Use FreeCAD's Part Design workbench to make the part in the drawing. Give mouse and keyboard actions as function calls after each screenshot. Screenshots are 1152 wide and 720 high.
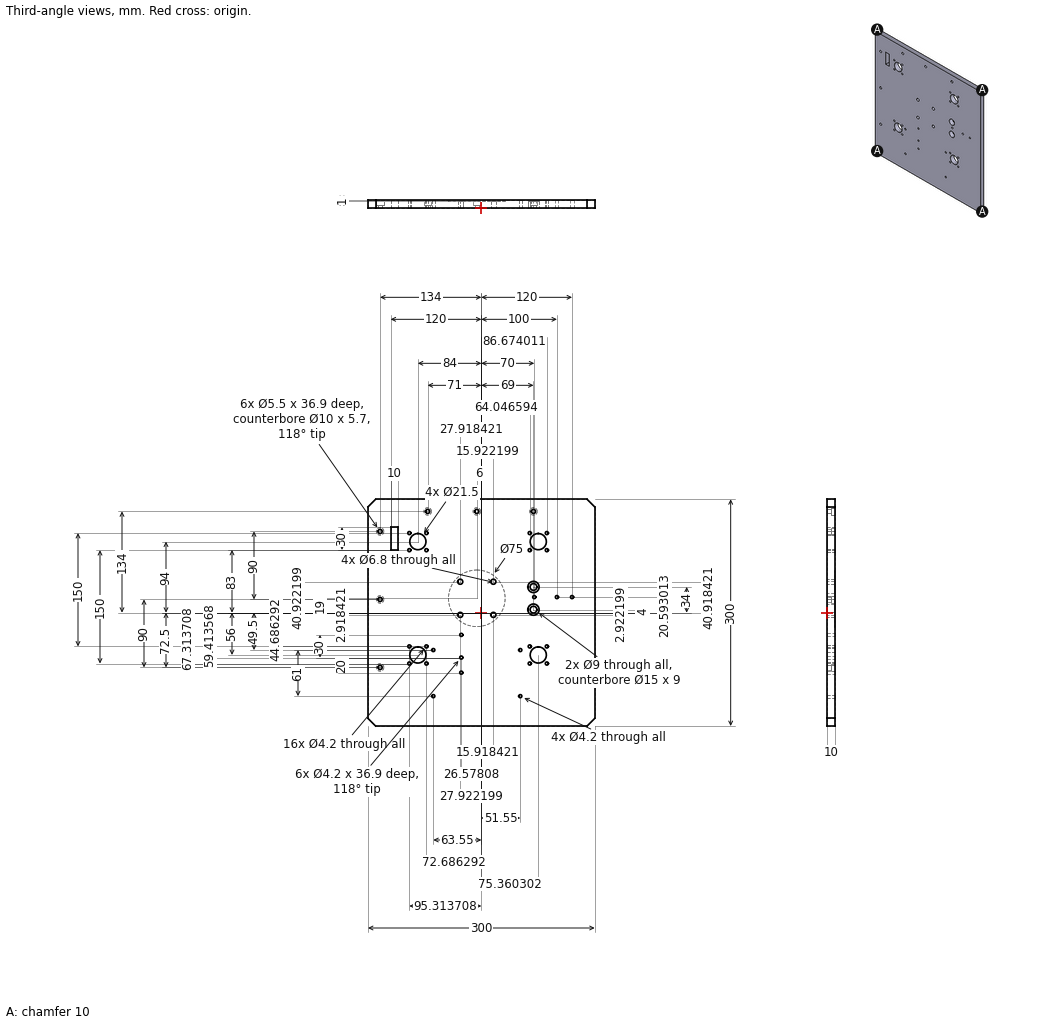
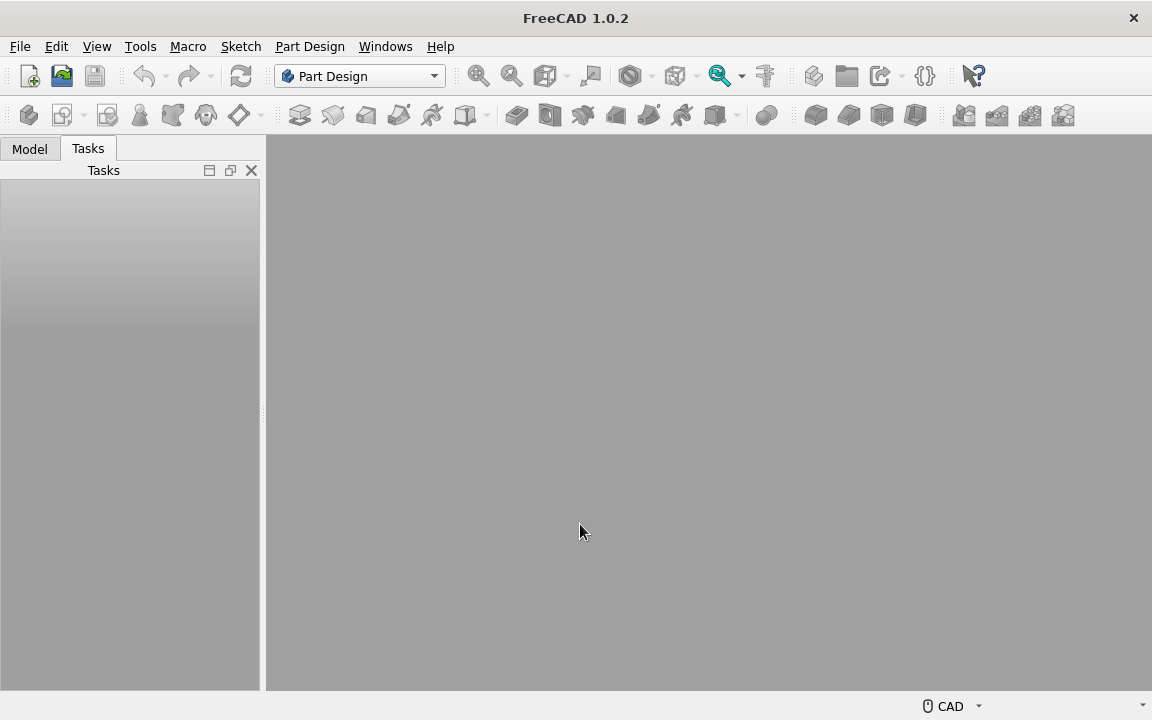
click(29, 76)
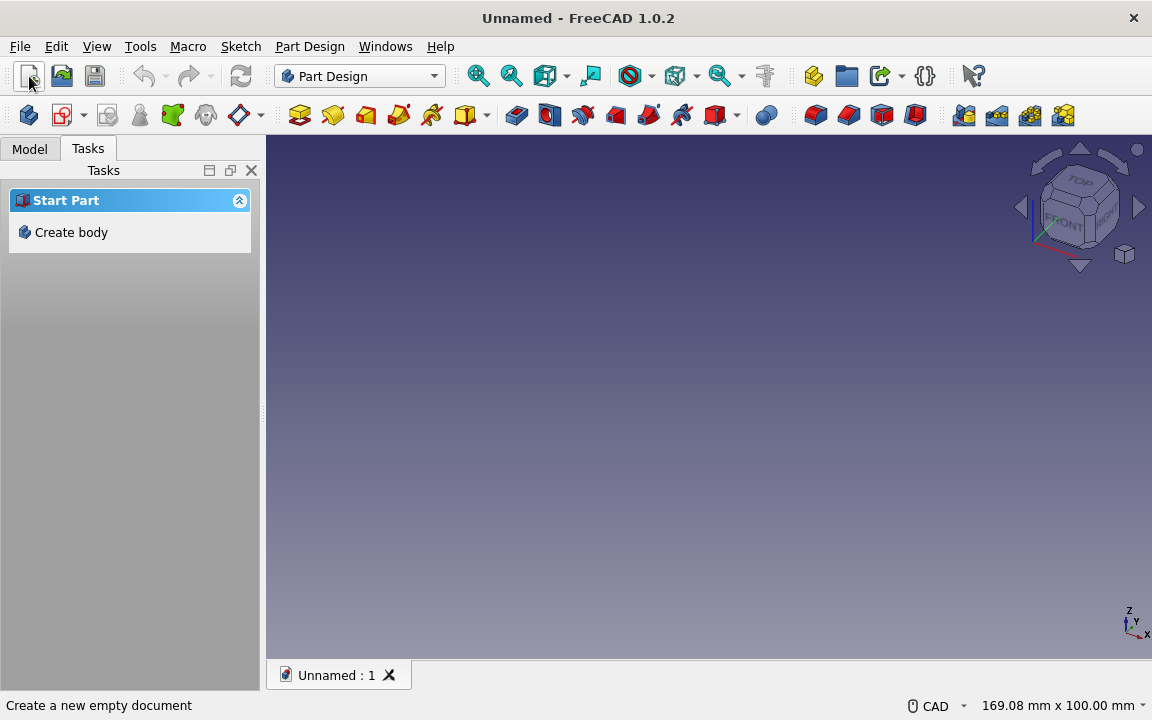
click(62, 116)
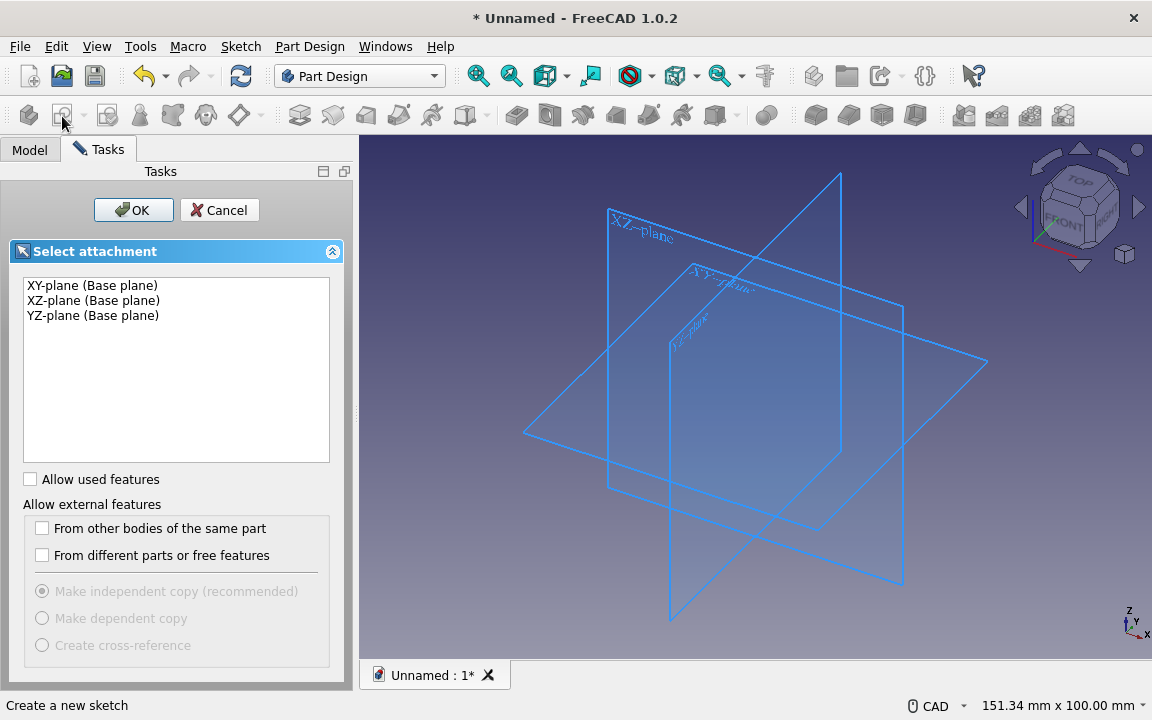
click(84, 300)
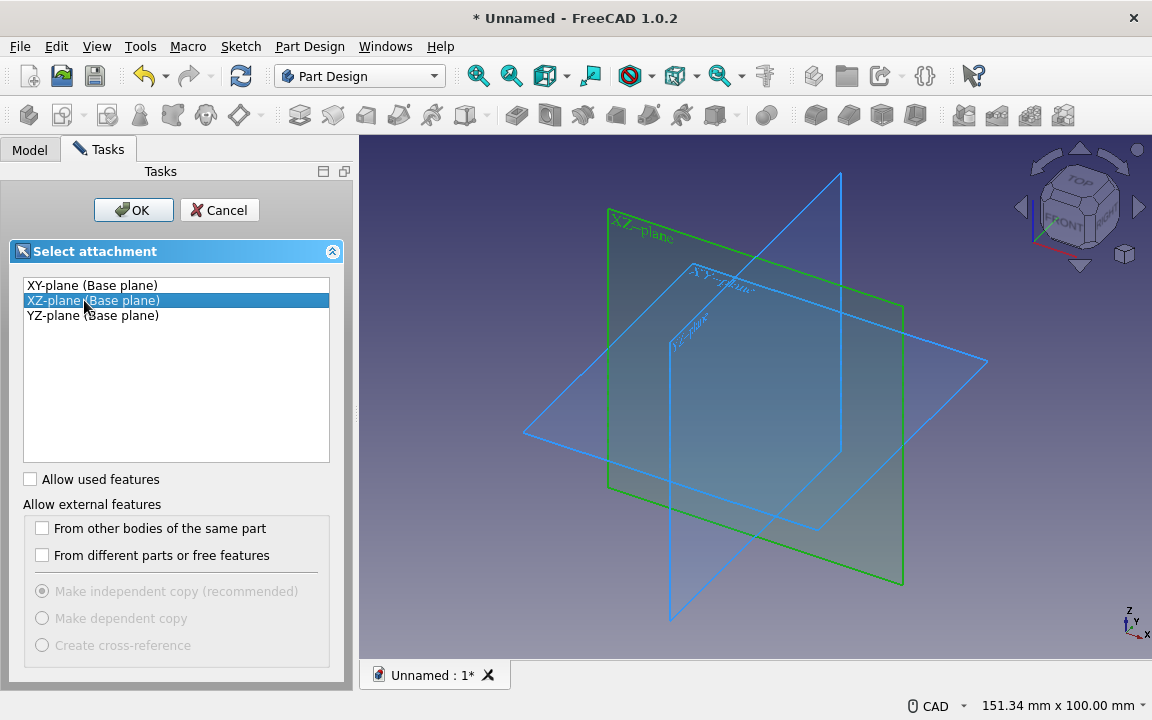
click(134, 210)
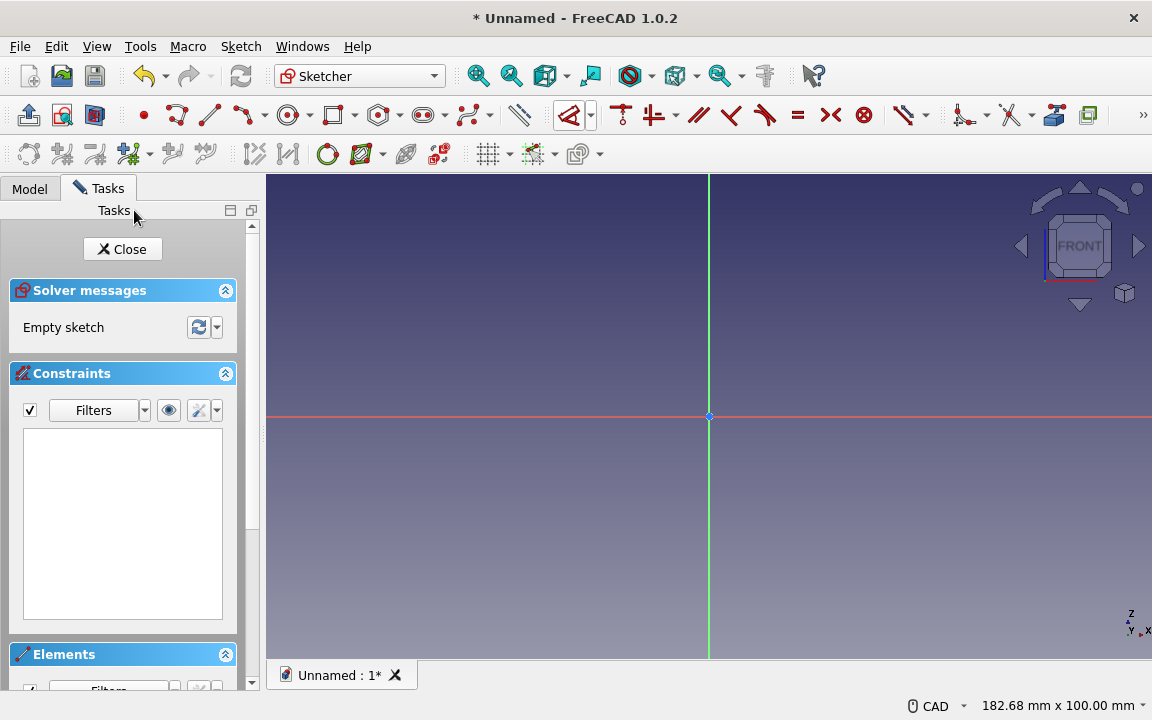
scroll(623, 416, down, 8)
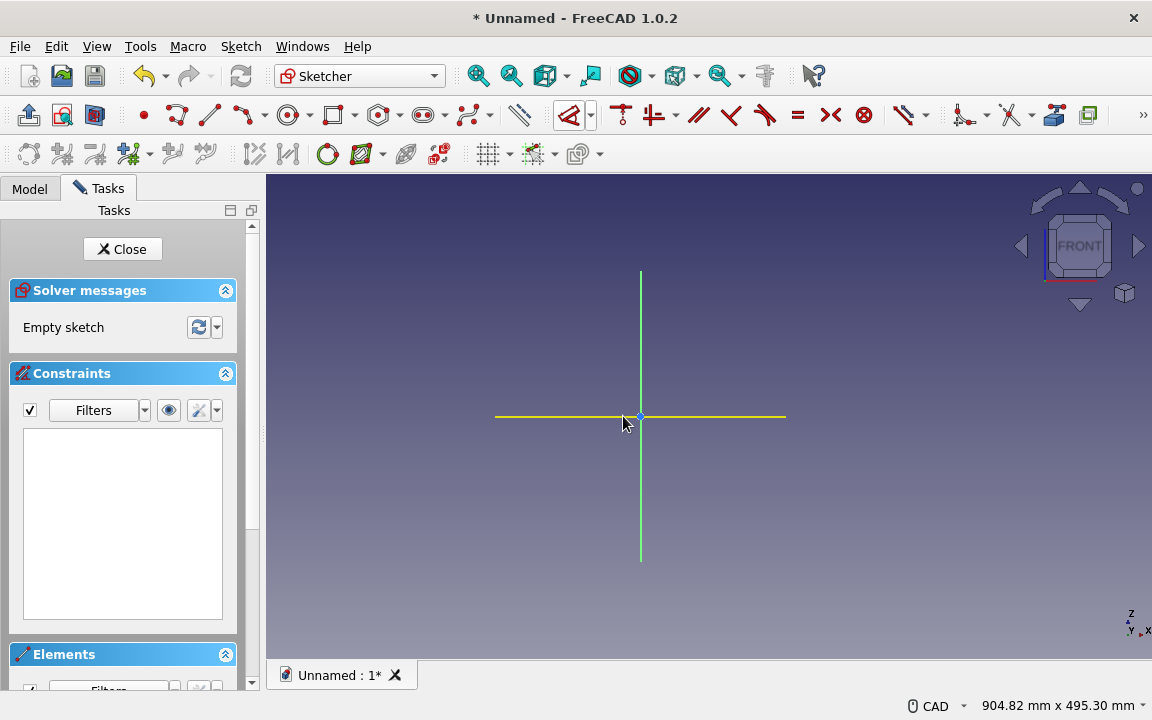
click(354, 116)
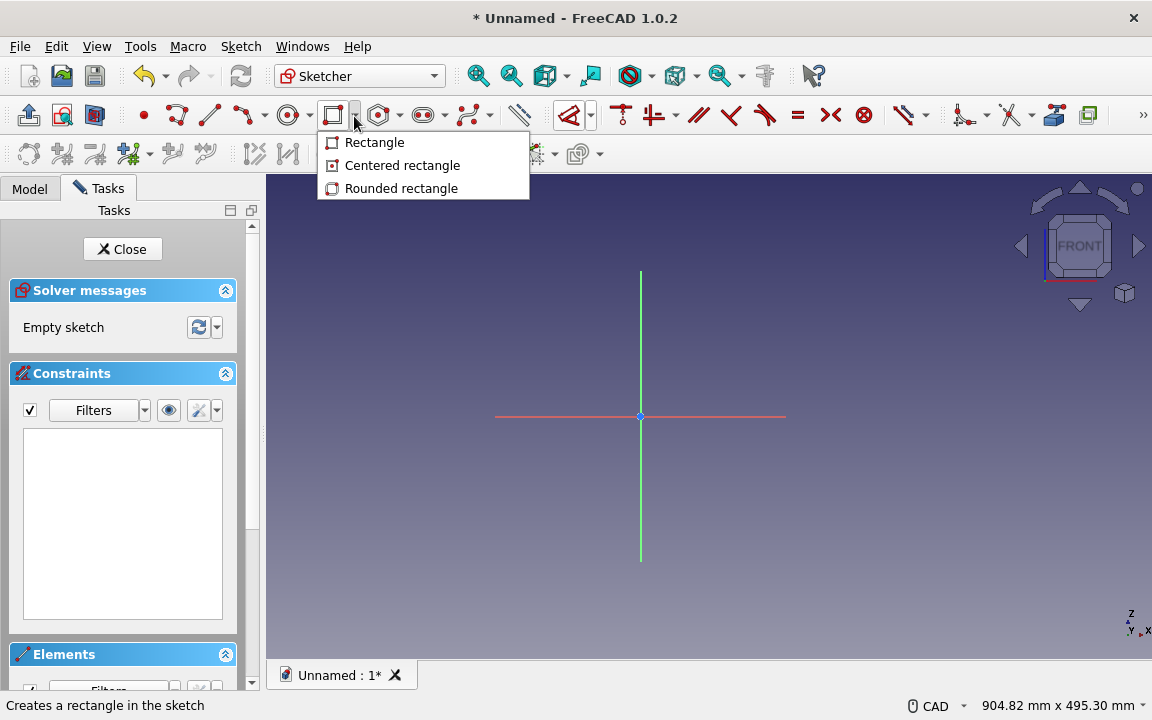
click(424, 166)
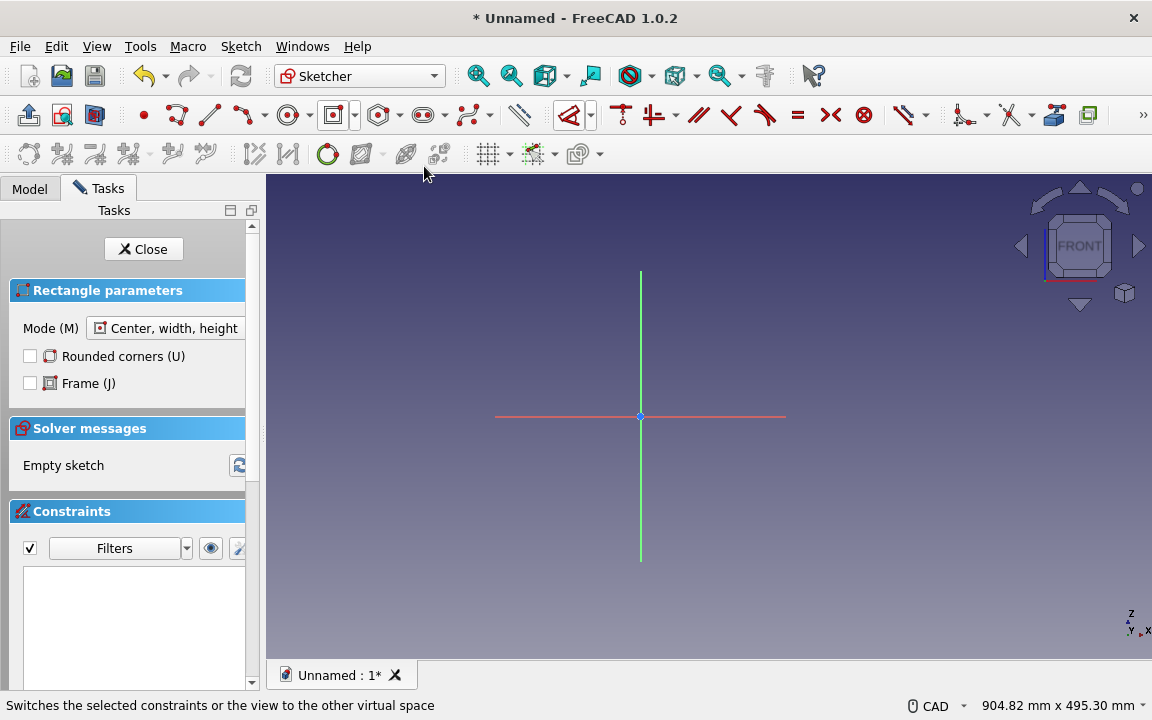
click(641, 416)
move(788, 270)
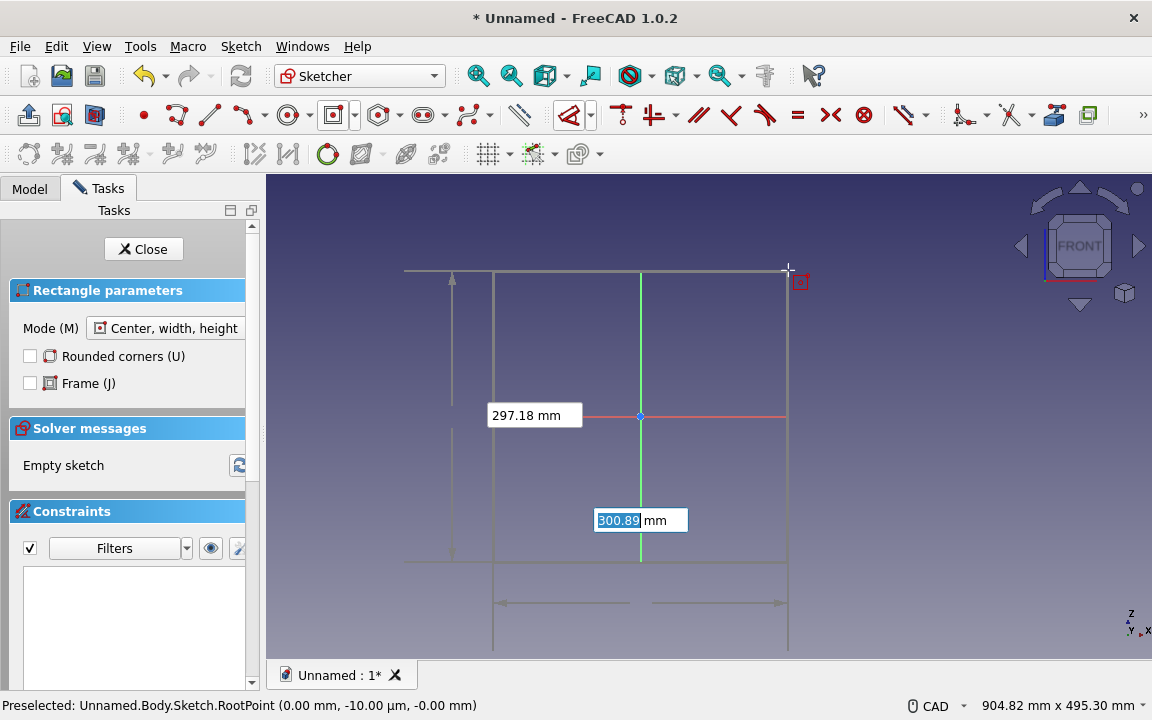
text(300)
key(Tab)
text(300)
key(Return)
key(Escape)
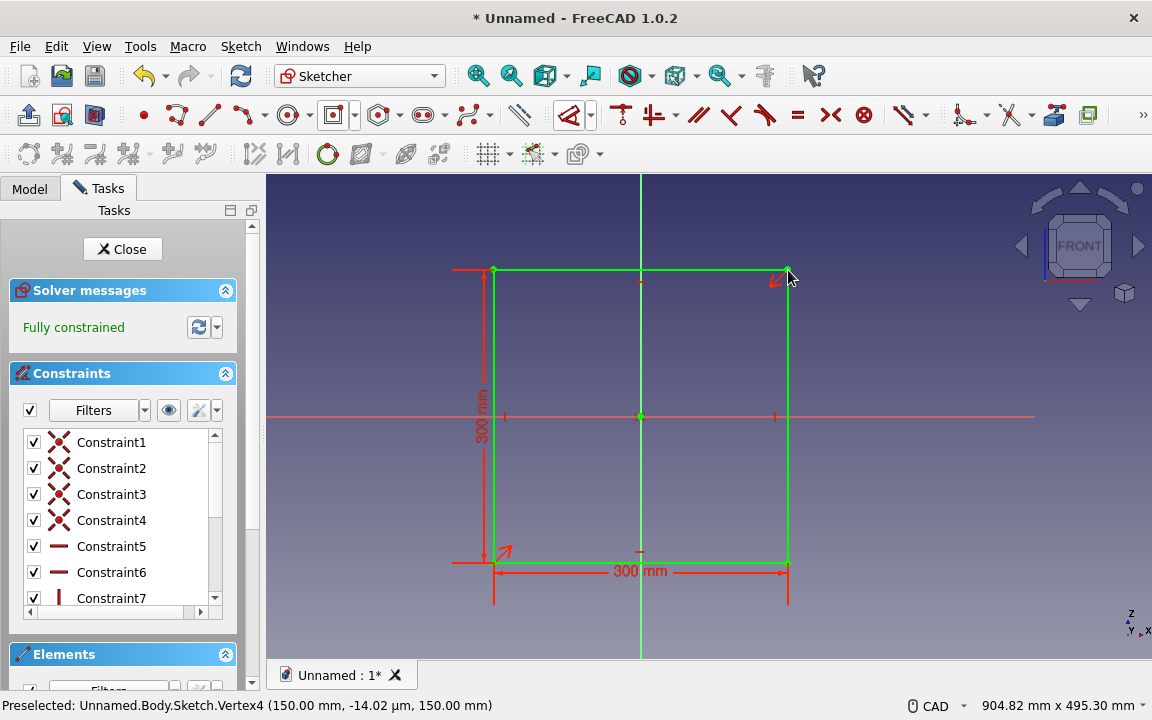
click(123, 249)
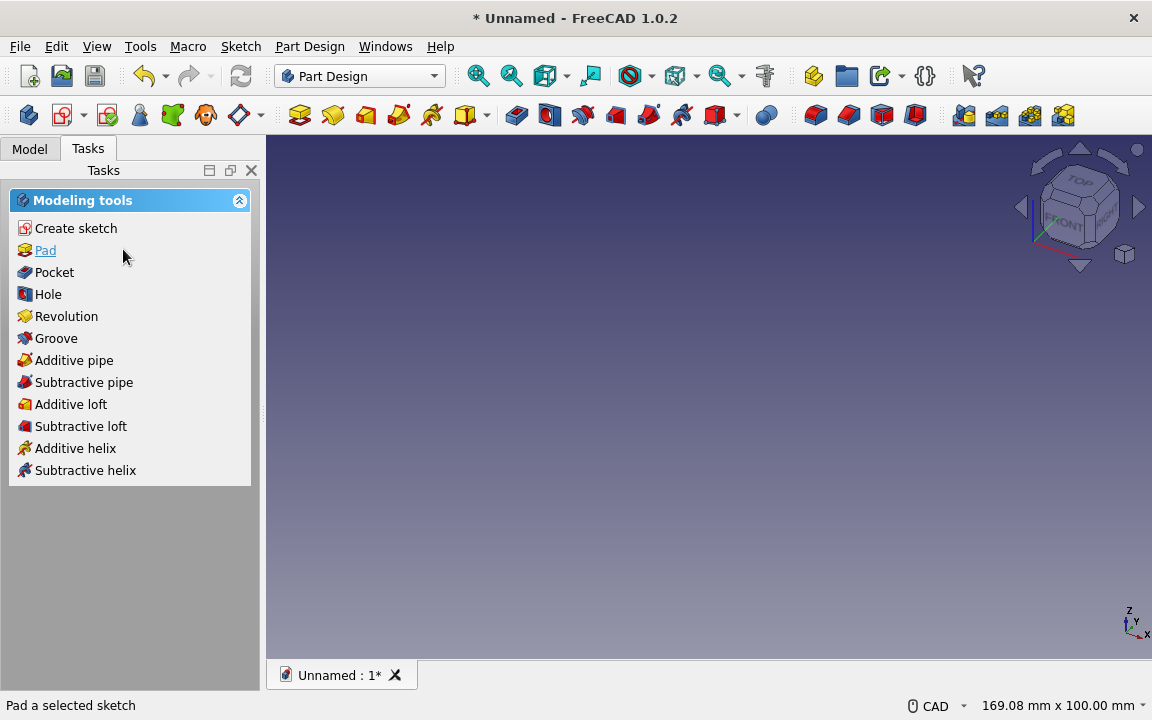
click(300, 116)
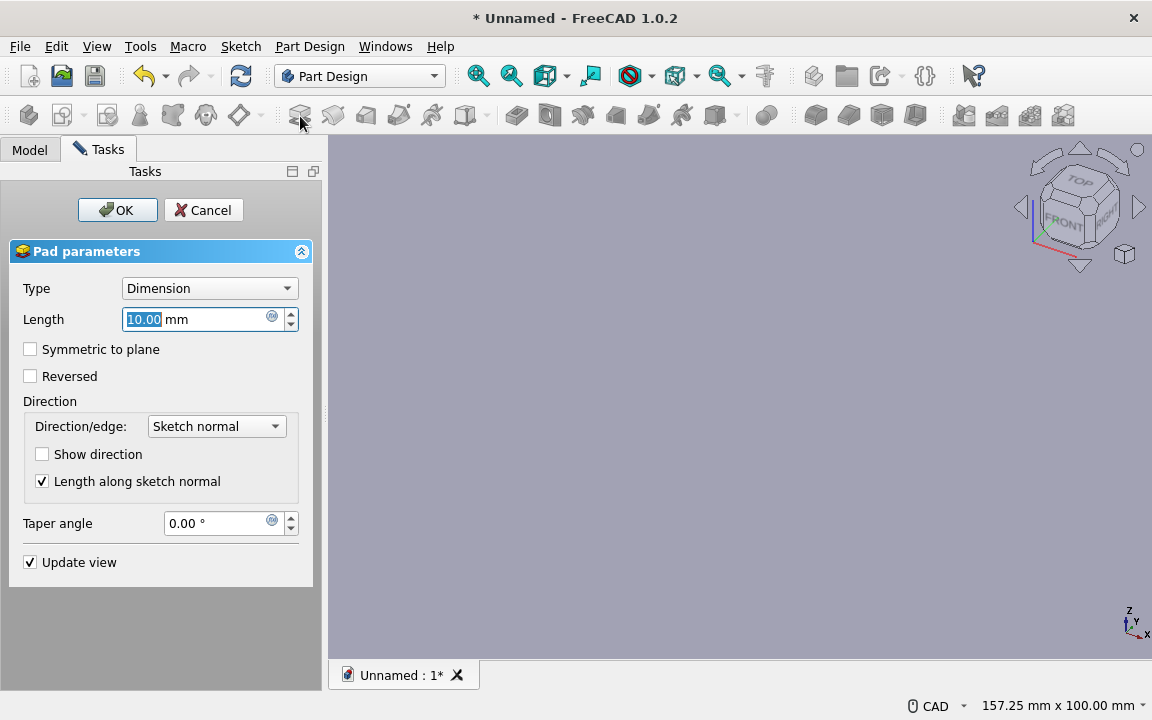
text(10)
key(Tab)